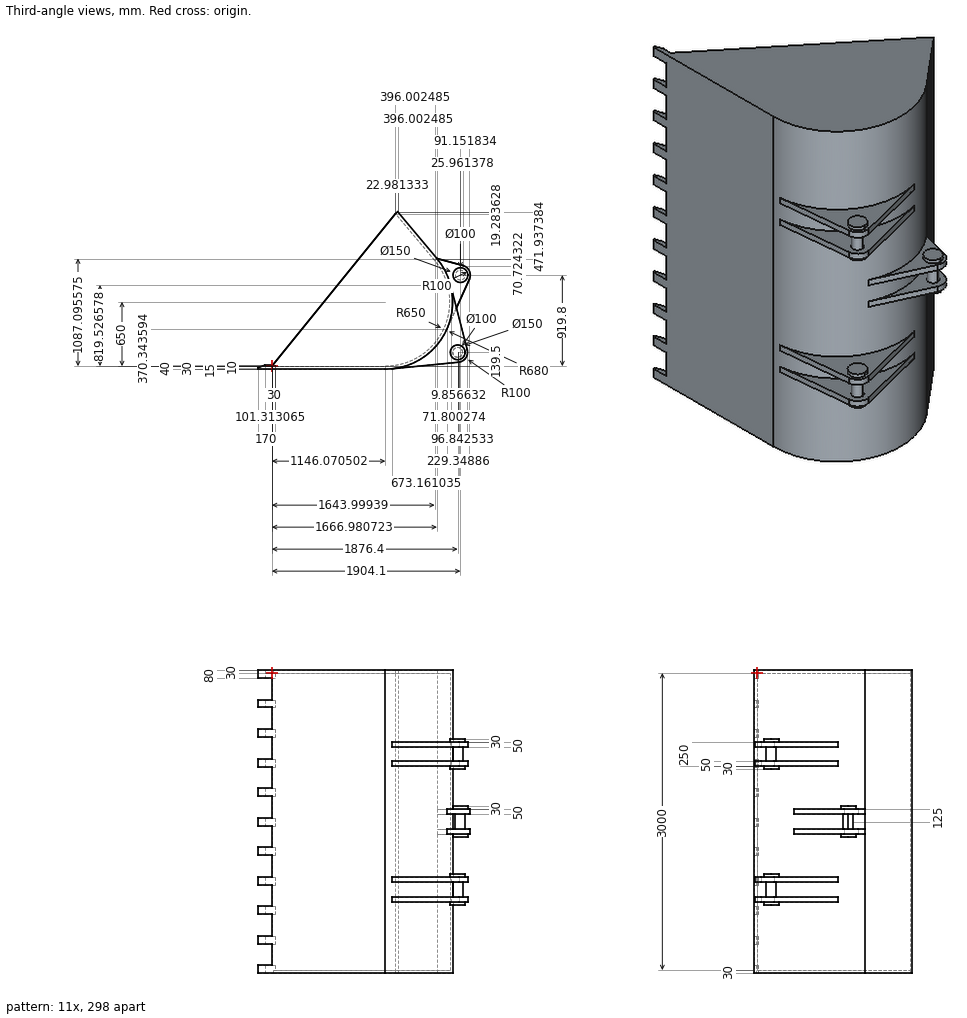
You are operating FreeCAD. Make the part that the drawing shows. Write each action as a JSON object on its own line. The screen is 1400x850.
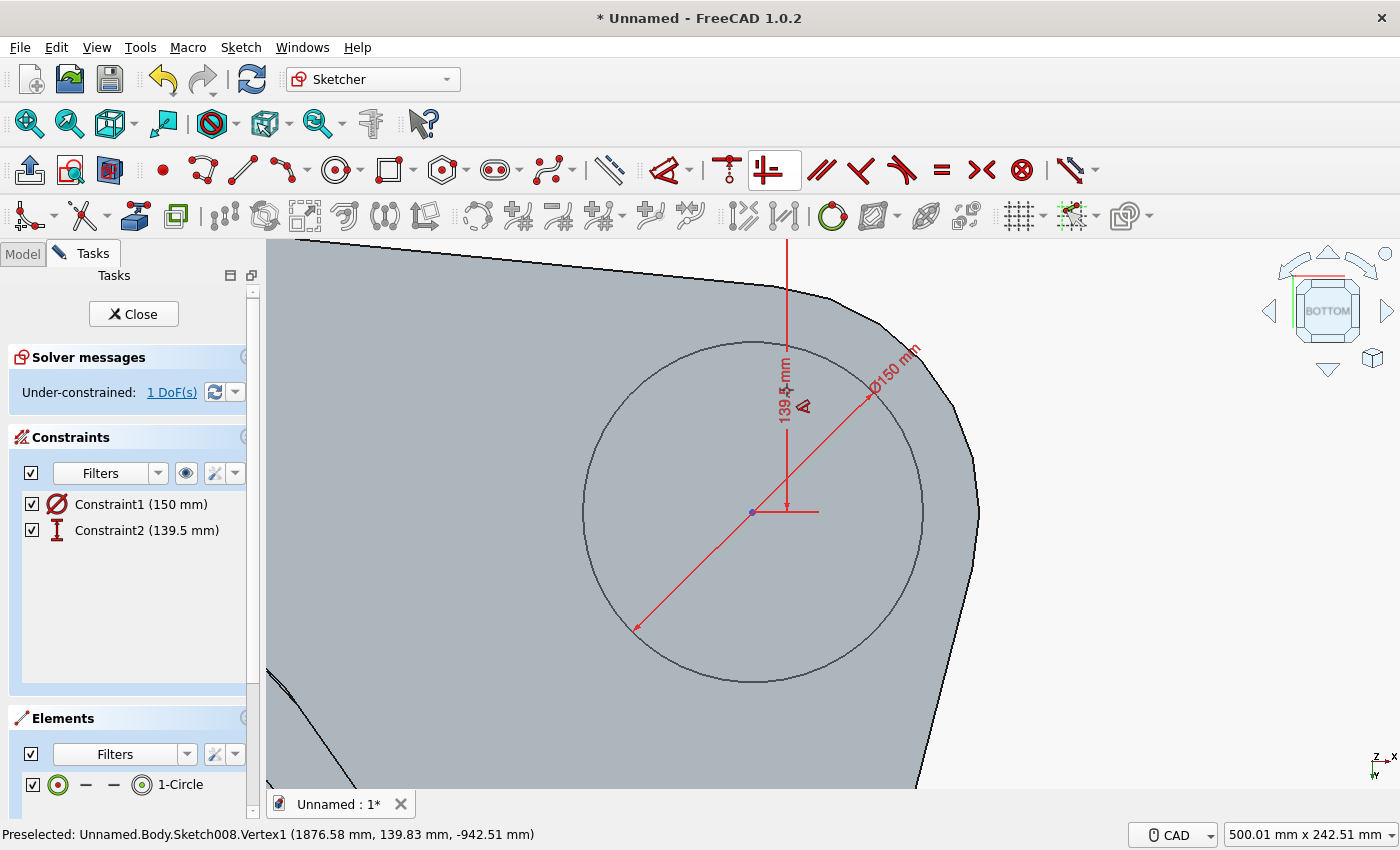
{"action": "left_click", "coordinate": [753, 512]}
{"action": "left_click", "coordinate": [523, 546]}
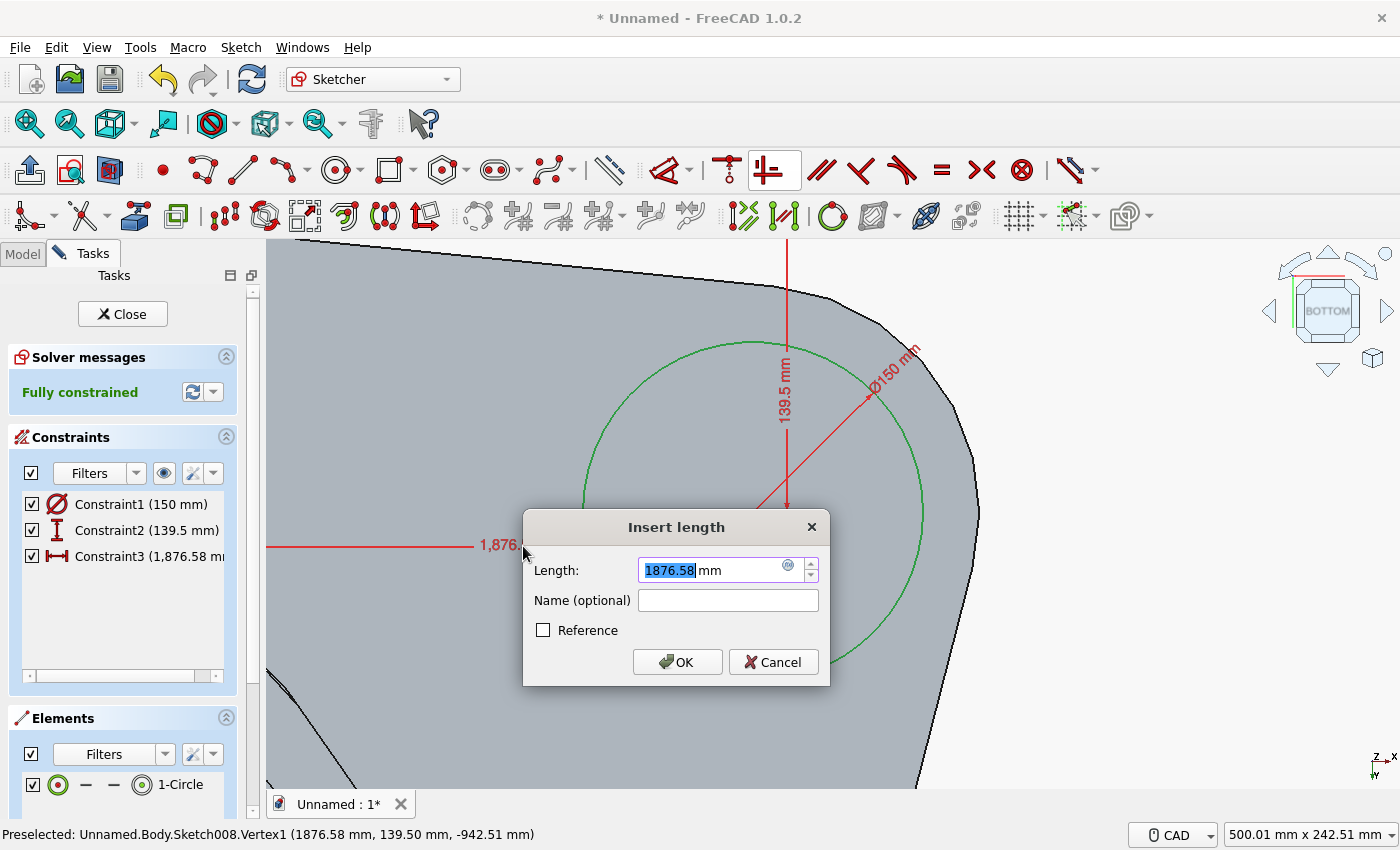
{"action": "type", "text": "1876.4"}
{"action": "key", "text": "Return"}
{"action": "key", "text": "Escape"}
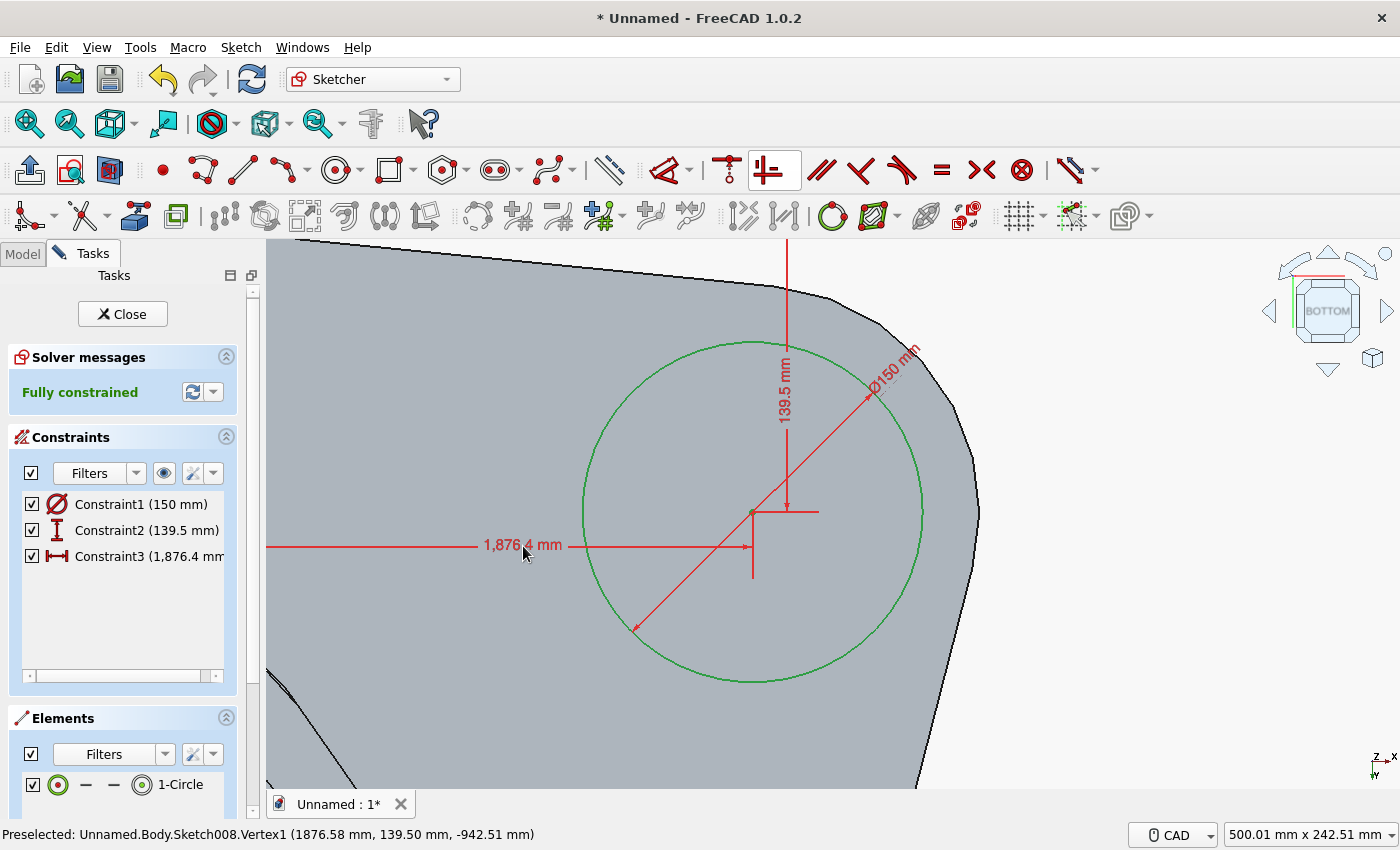
{"action": "left_click", "coordinate": [123, 314]}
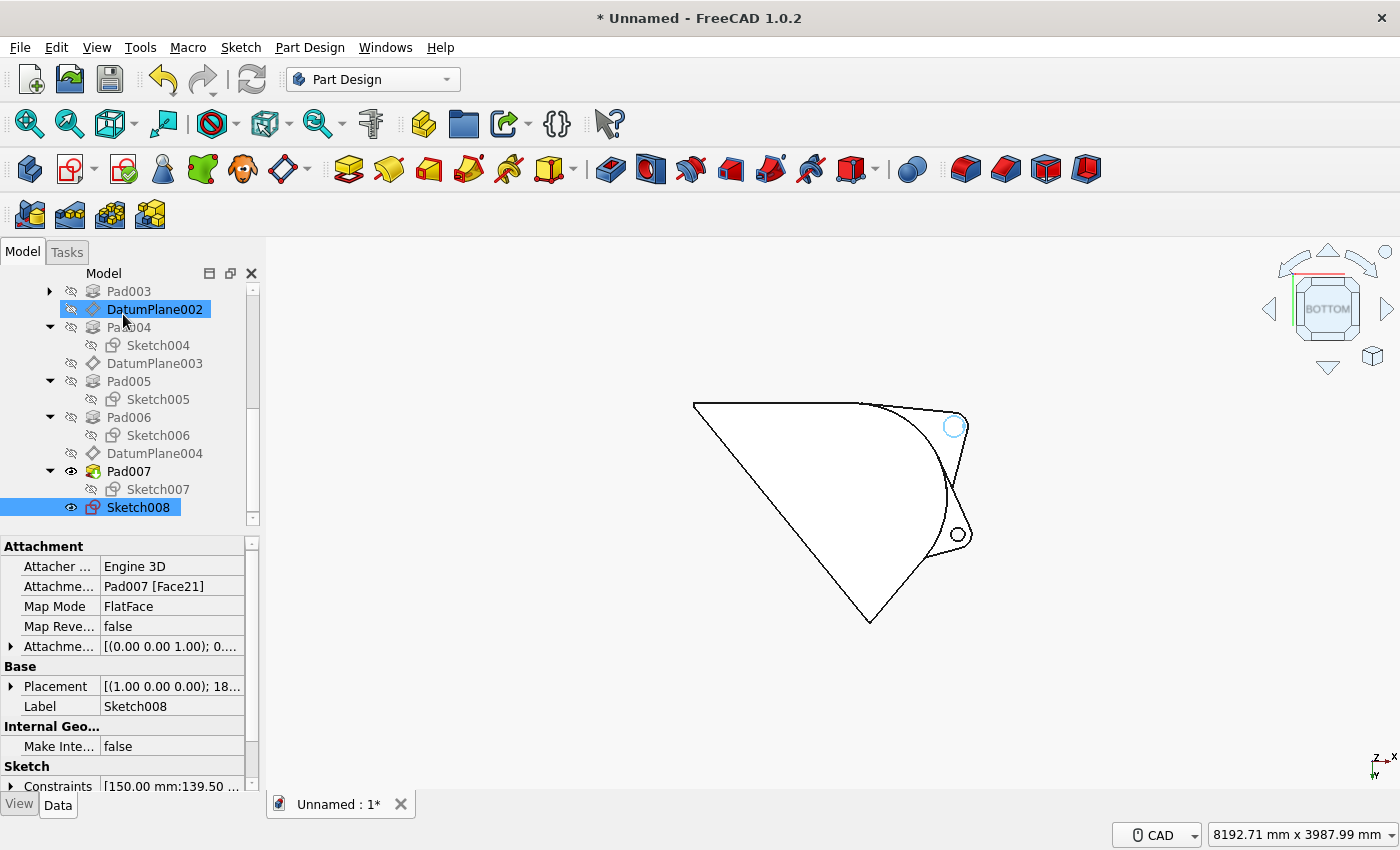
{"action": "left_click", "coordinate": [350, 170]}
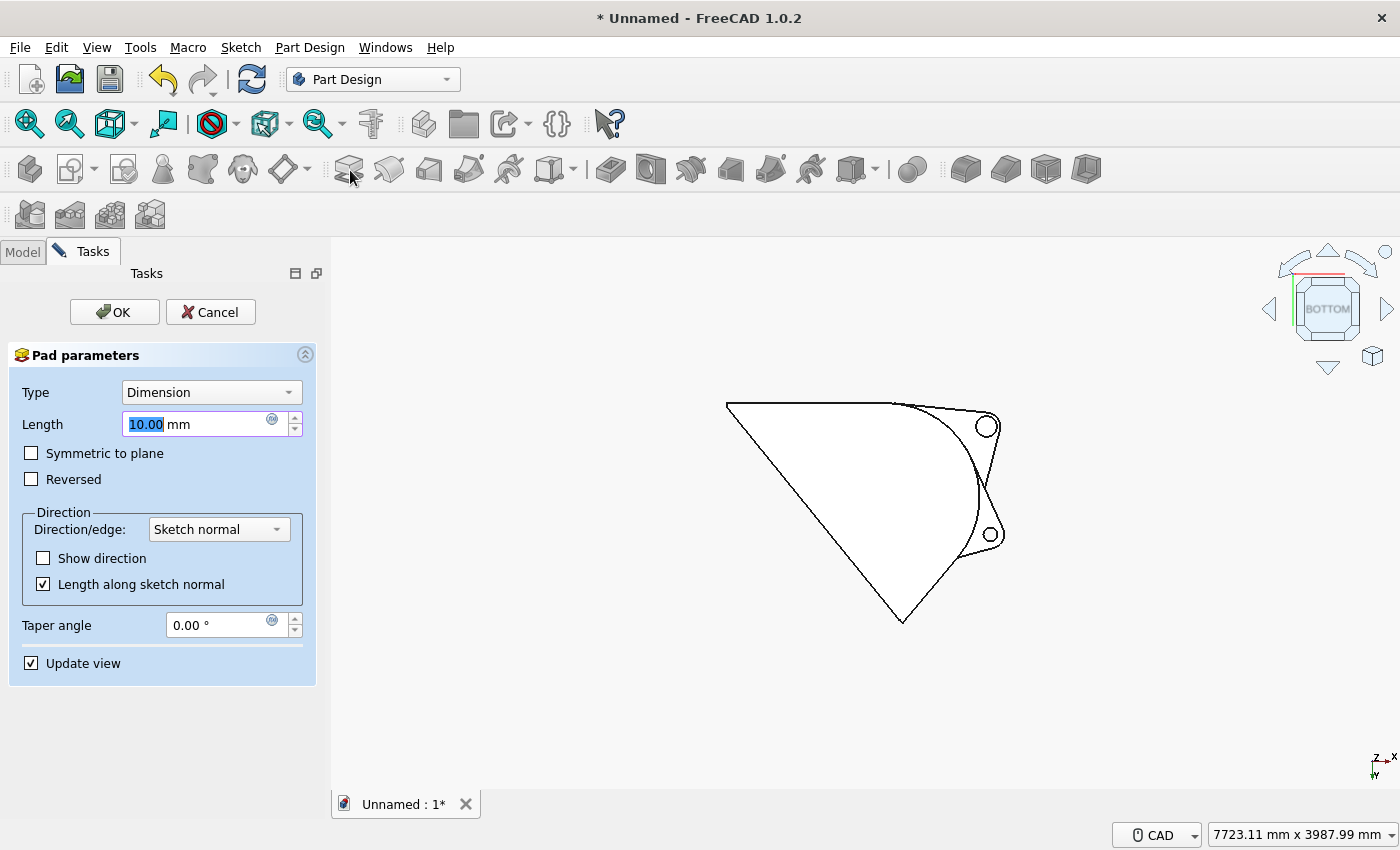
{"action": "type", "text": "30"}
{"action": "key", "text": "Tab"}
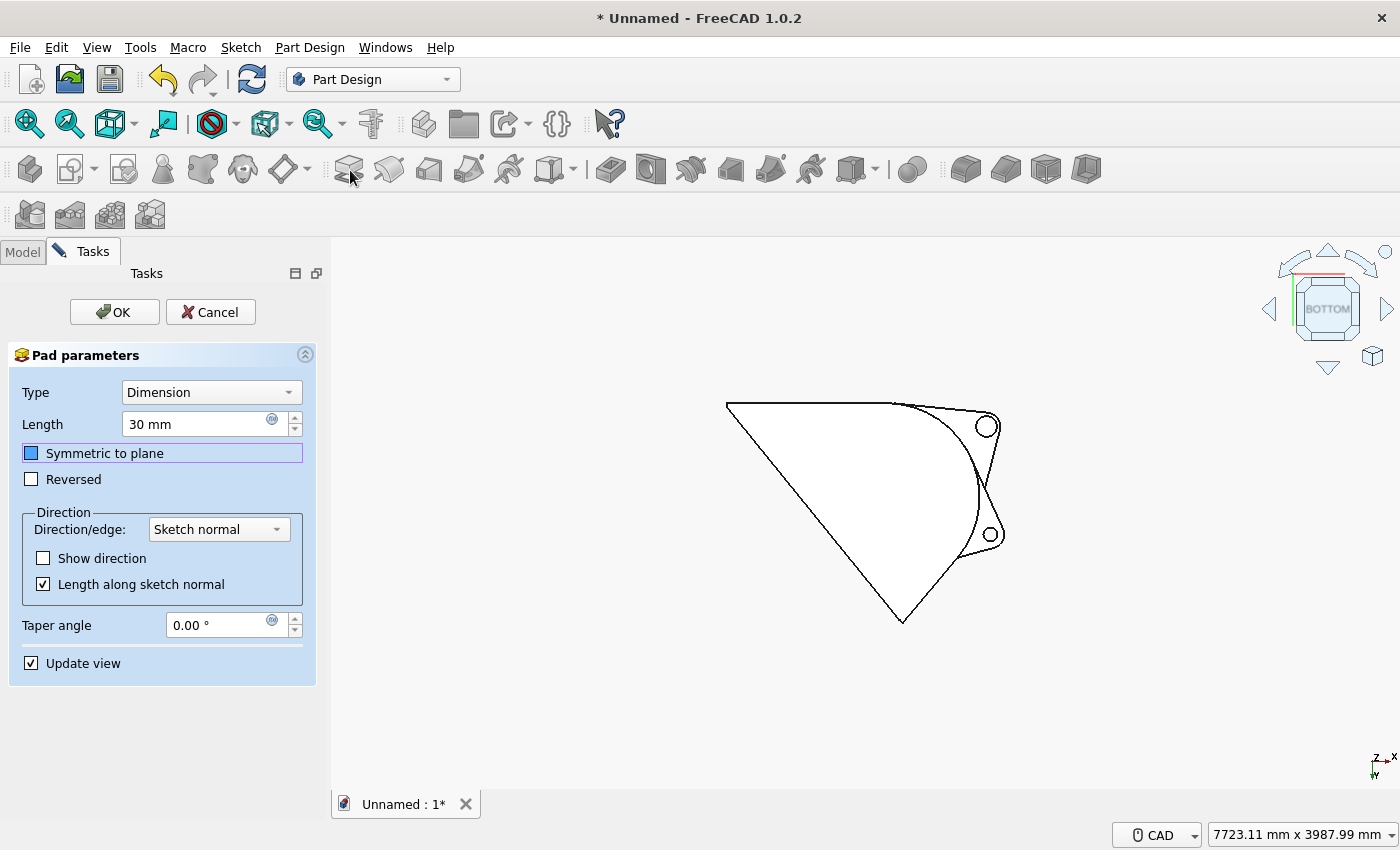
{"action": "left_click", "coordinate": [115, 312]}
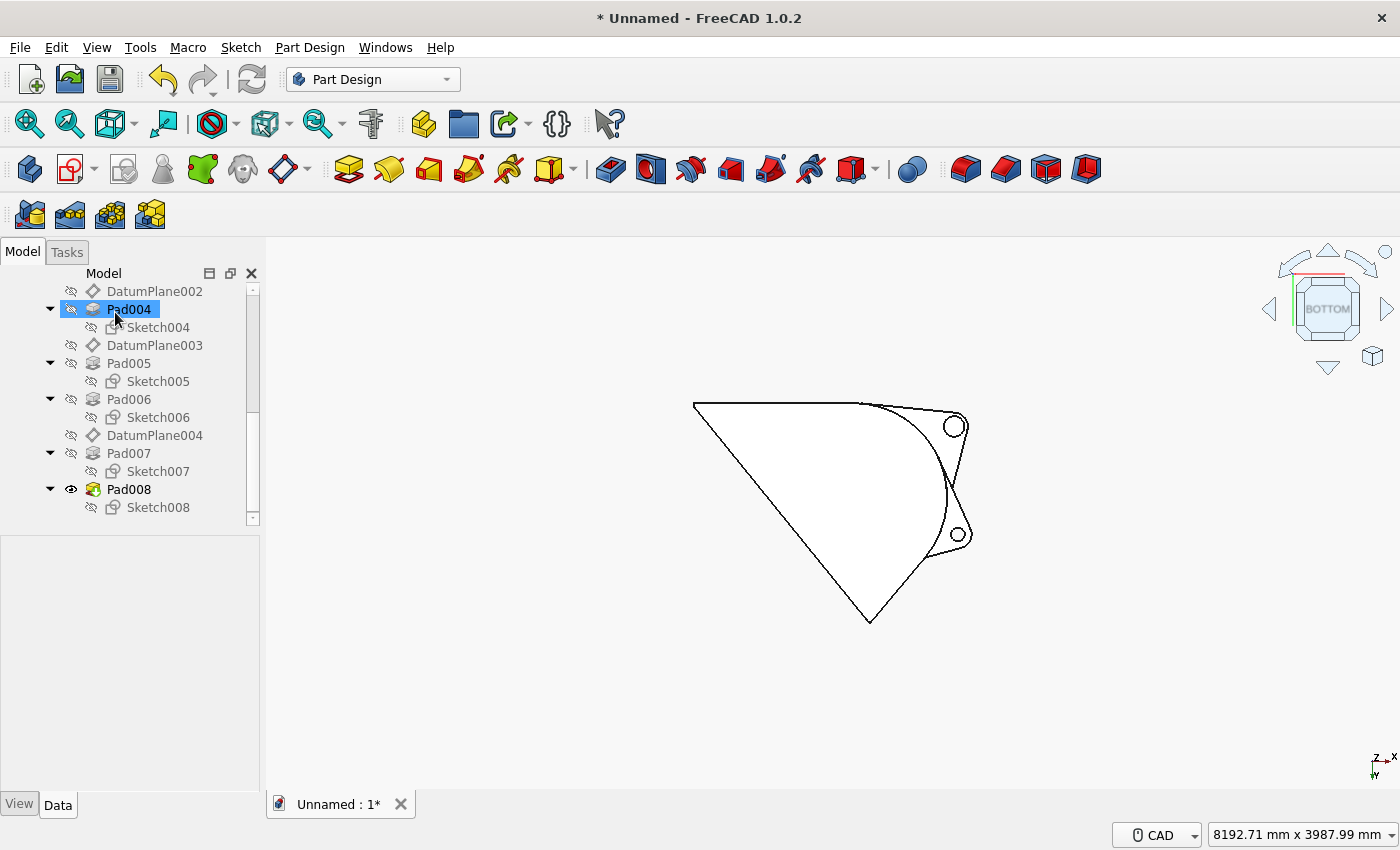
{"action": "key", "text": "v f"}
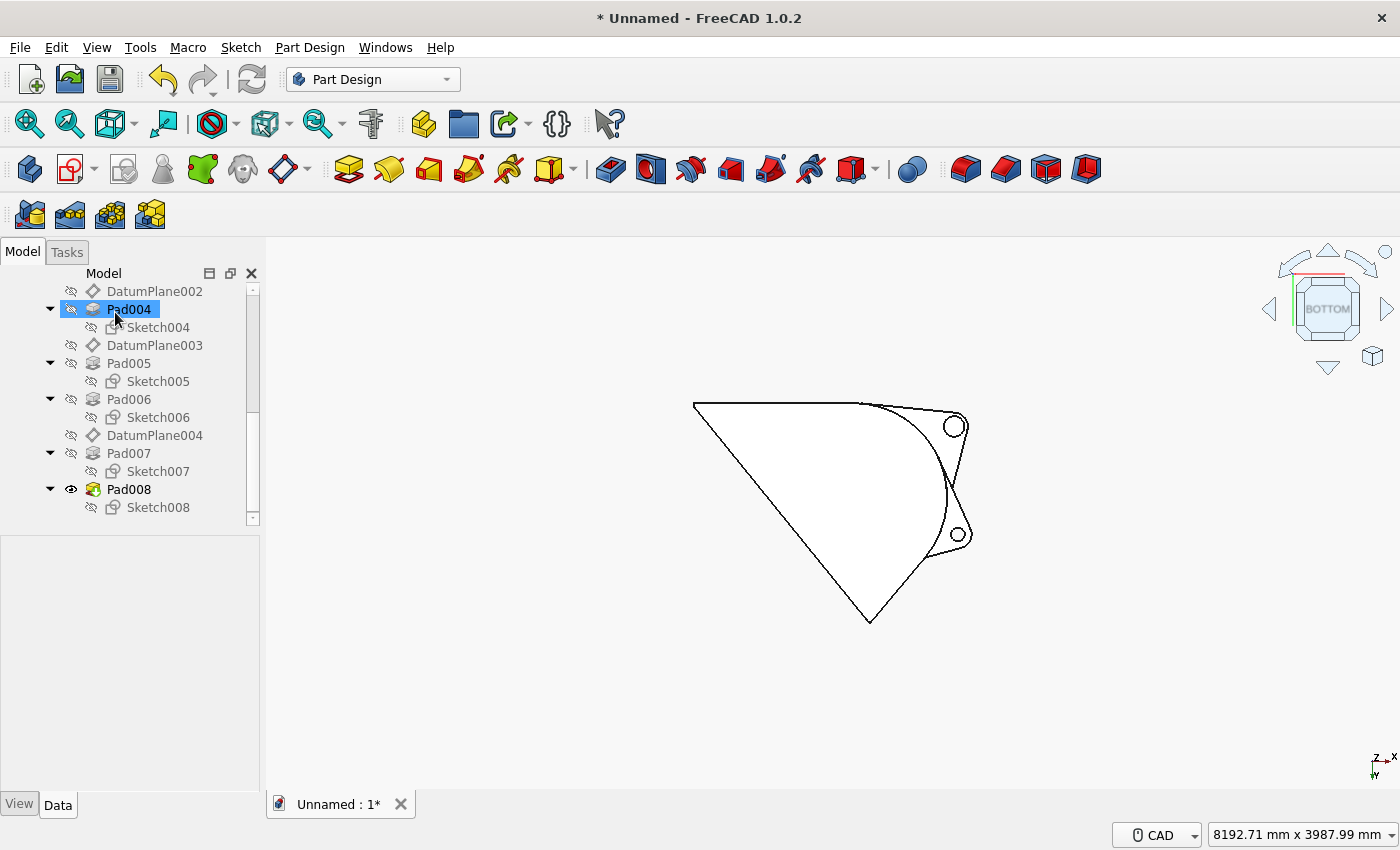
{"action": "scroll", "coordinate": [140, 395], "scroll_direction": "down", "scroll_amount": 3}